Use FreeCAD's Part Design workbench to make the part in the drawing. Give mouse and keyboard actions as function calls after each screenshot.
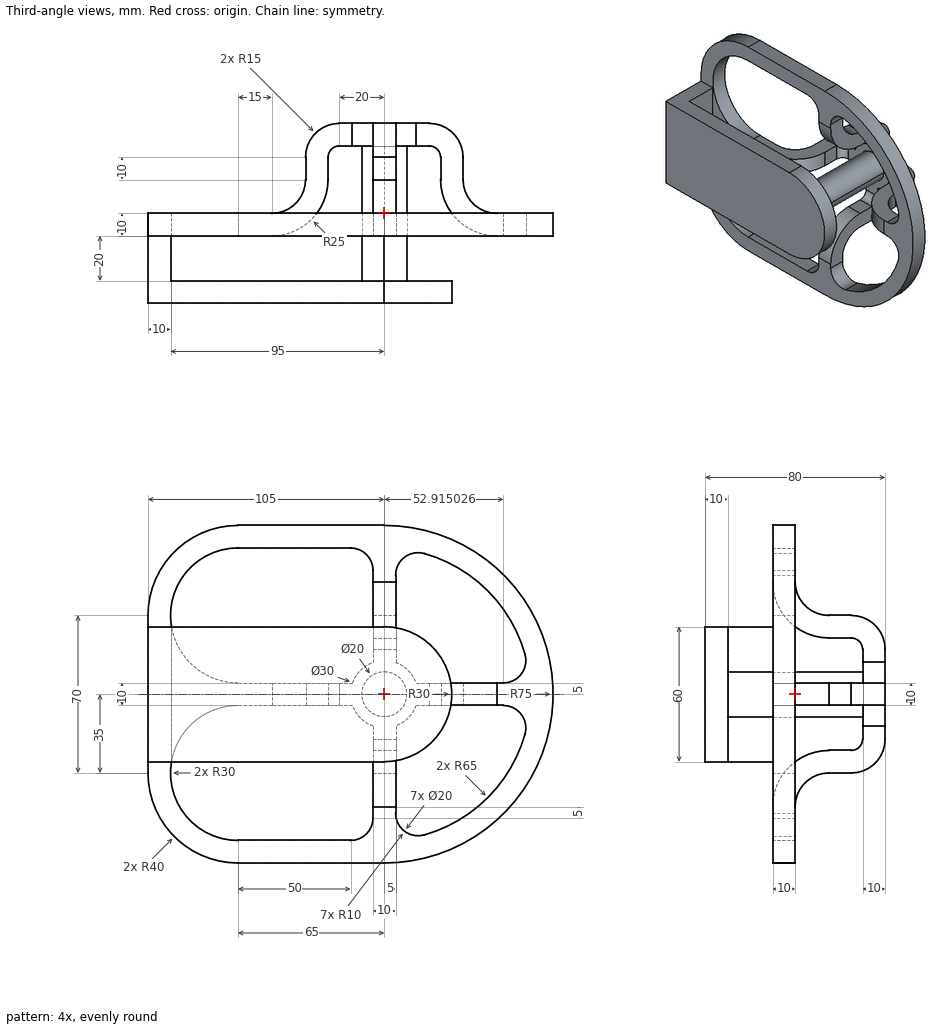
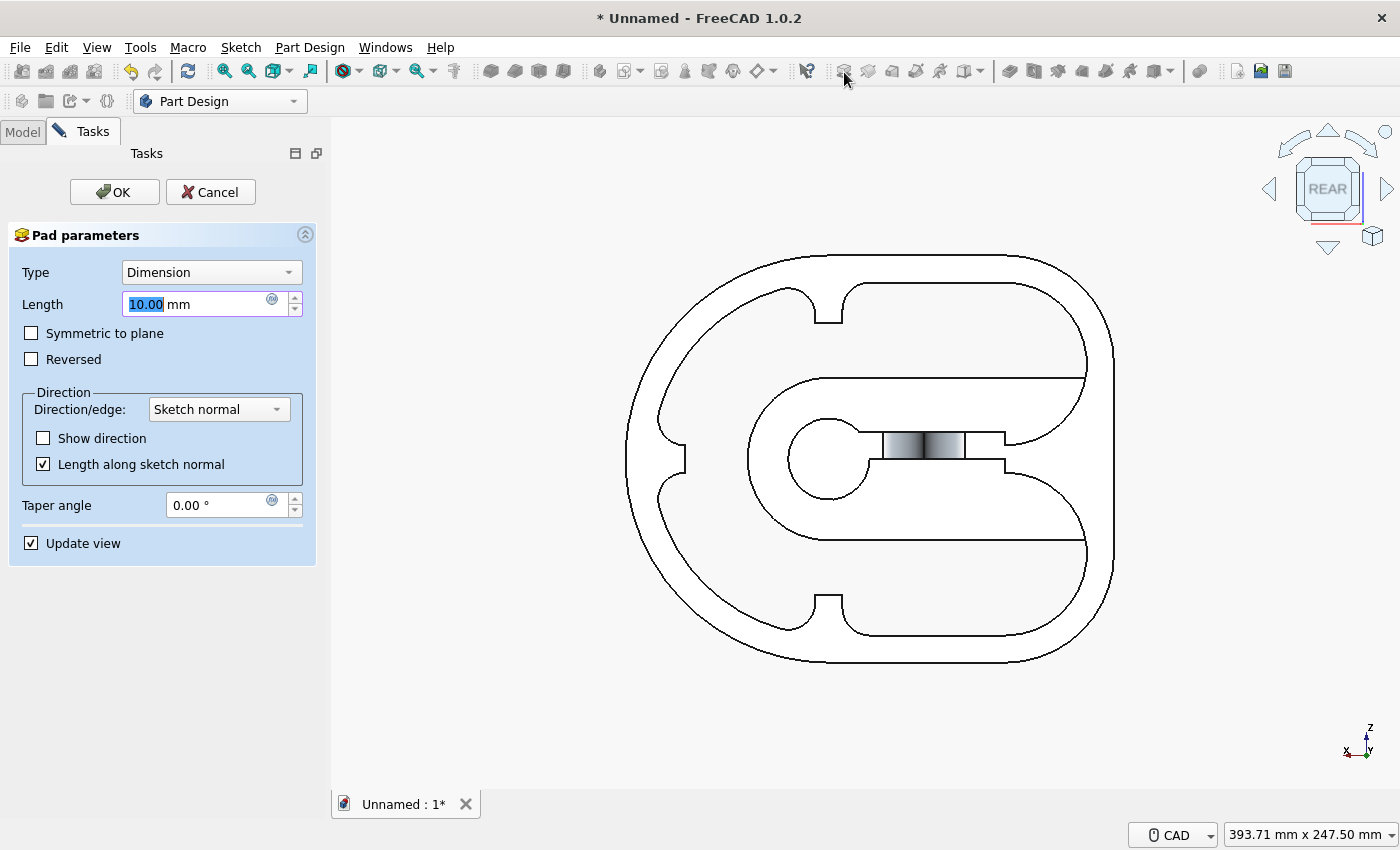
text(10)
key(Tab)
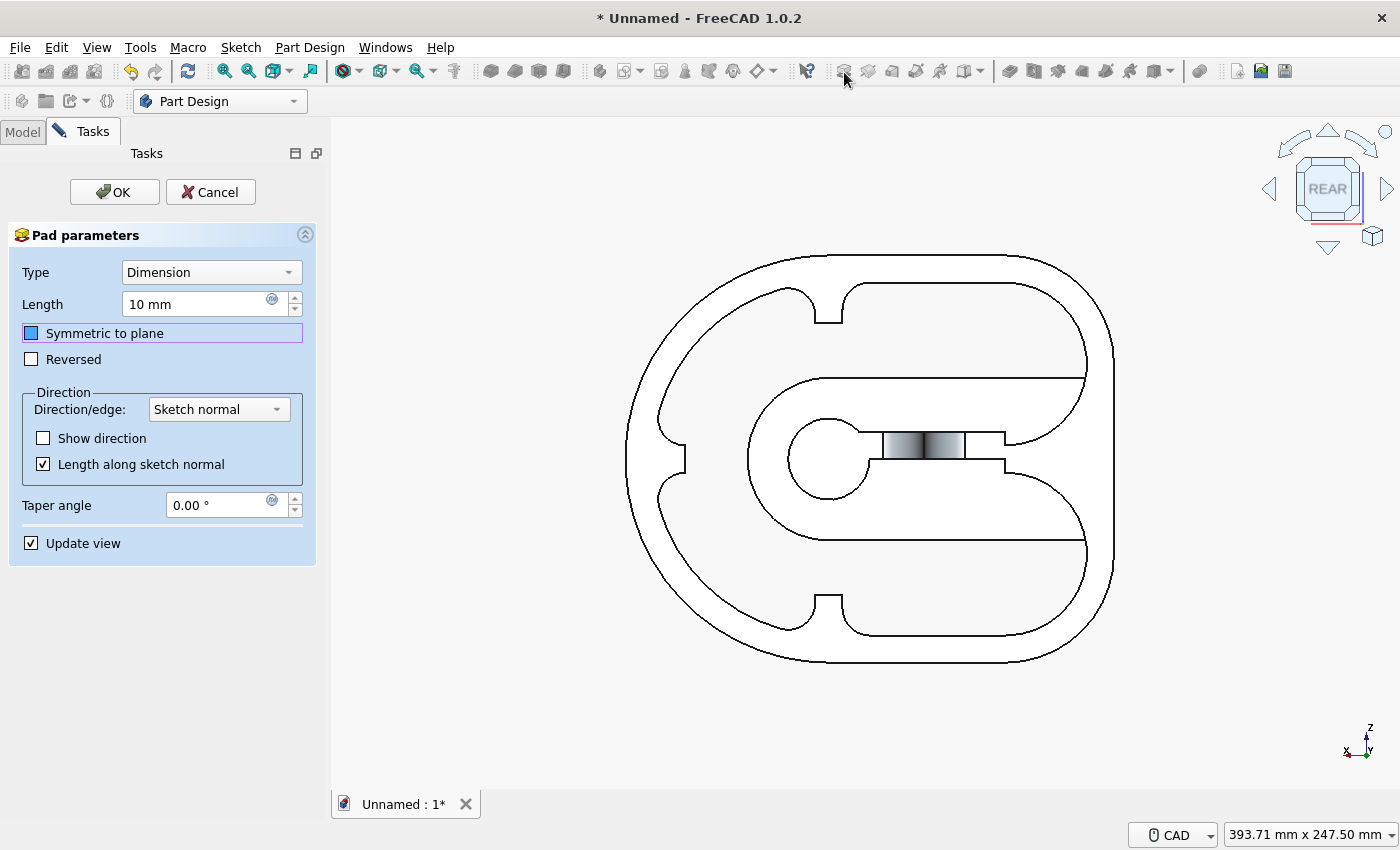
click(30, 333)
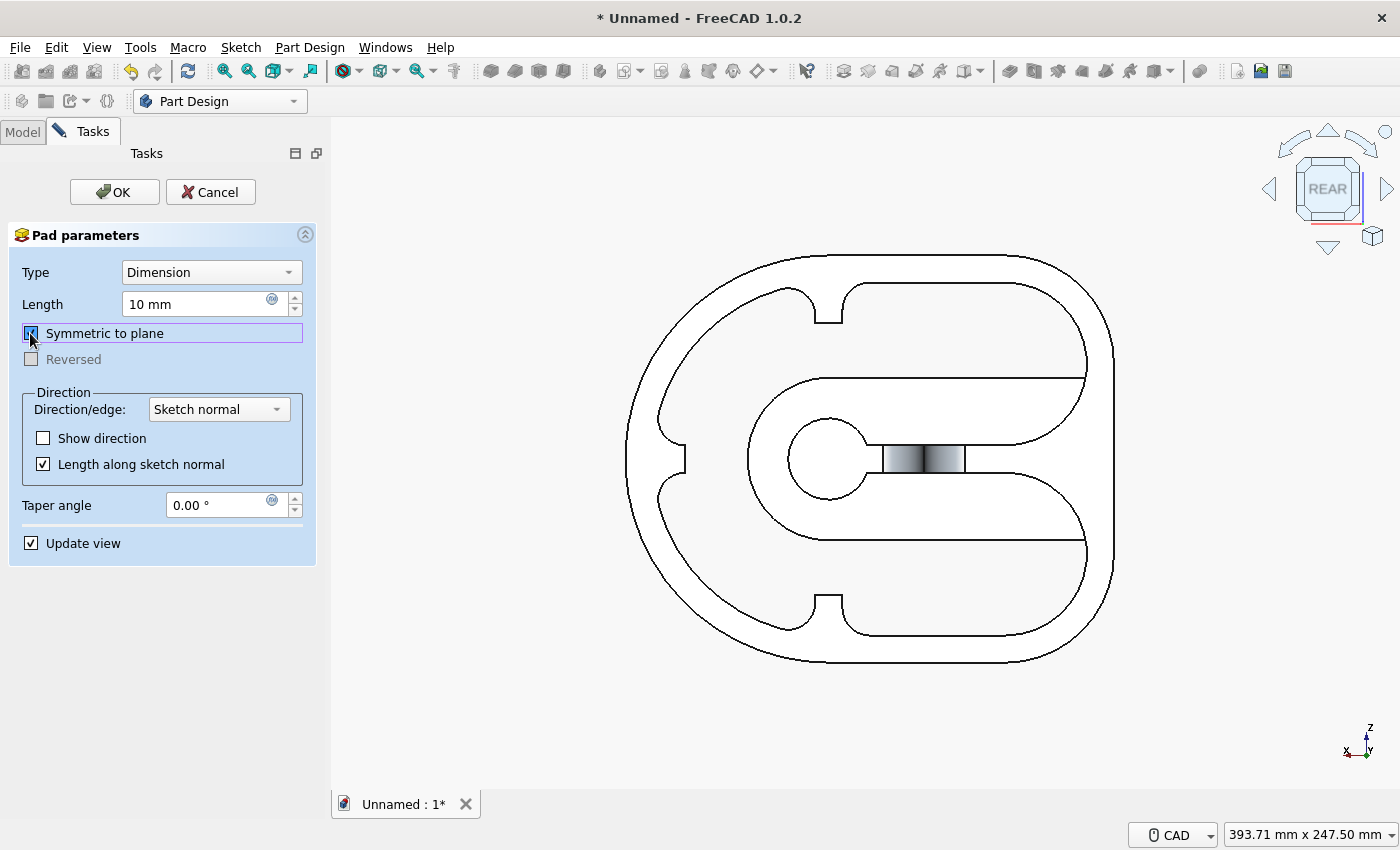
click(115, 192)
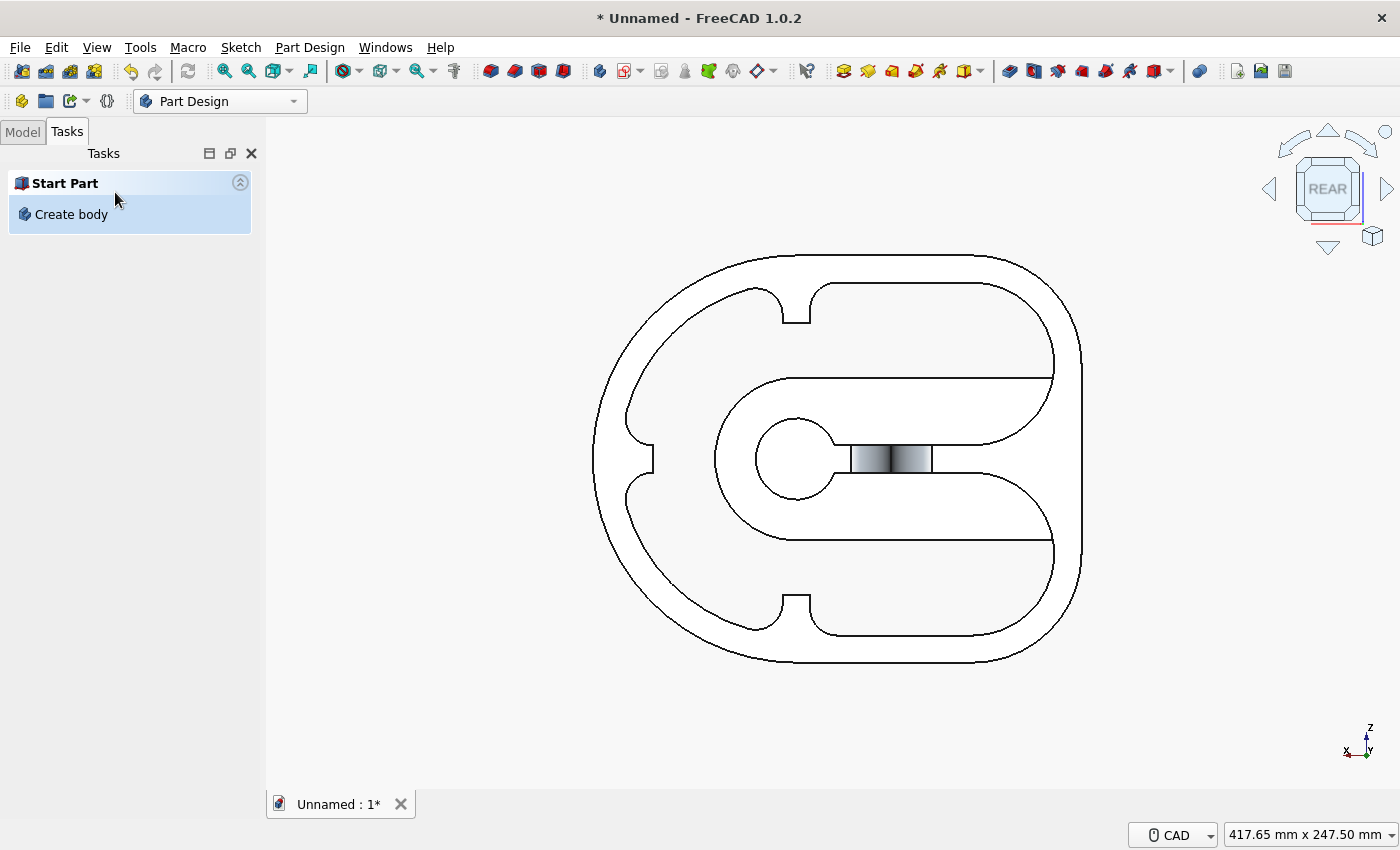
click(23, 131)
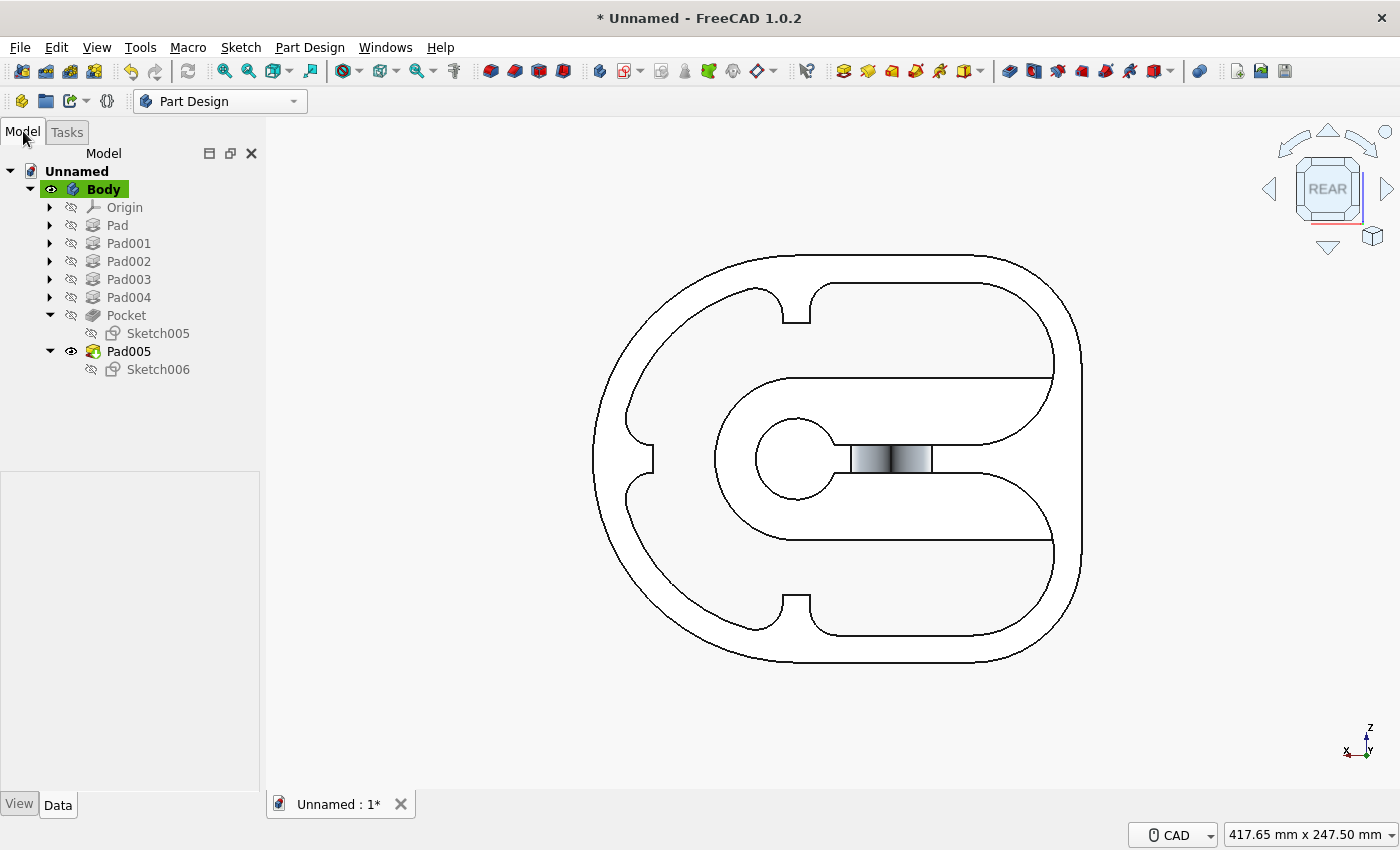
click(116, 351)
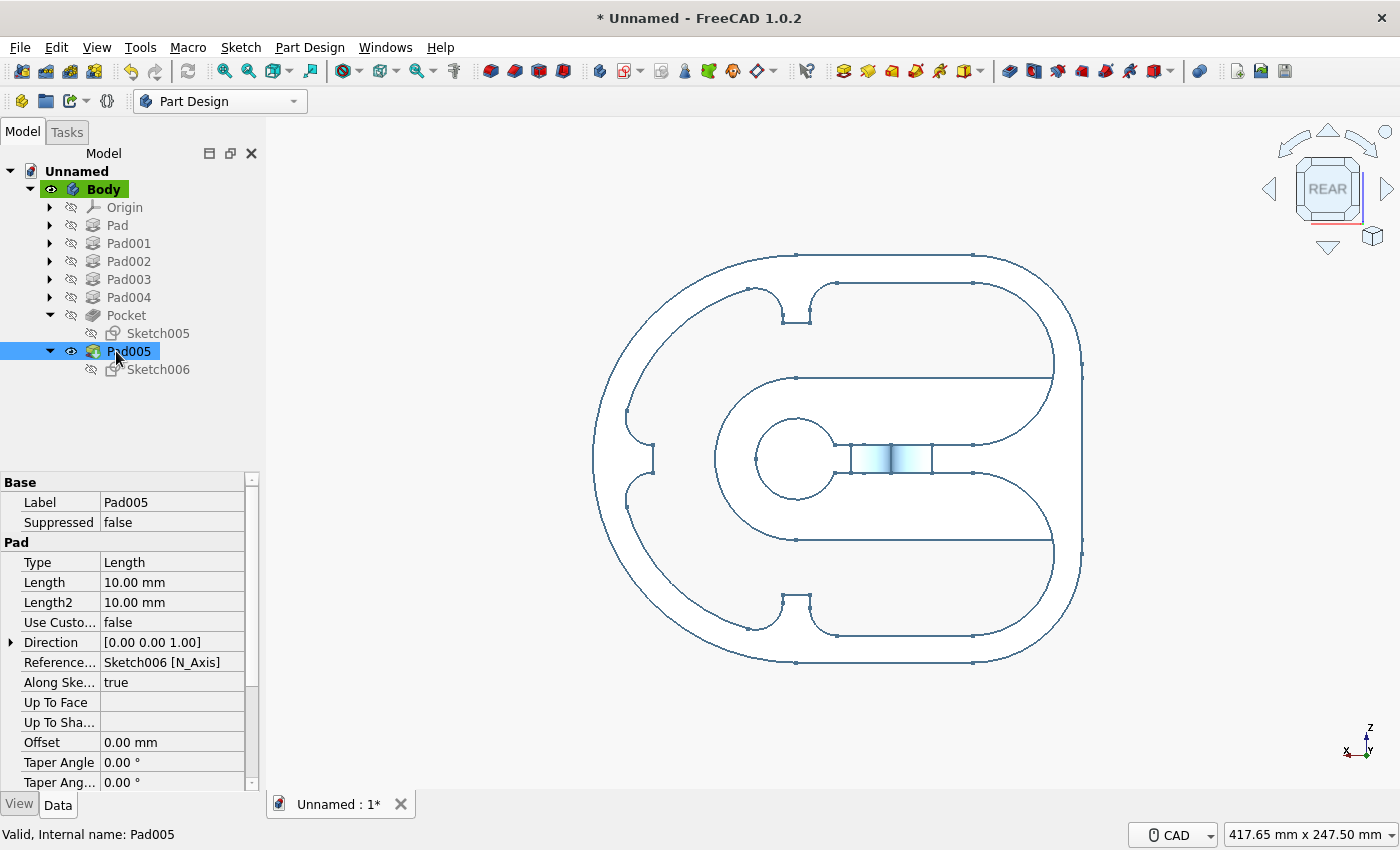
click(70, 72)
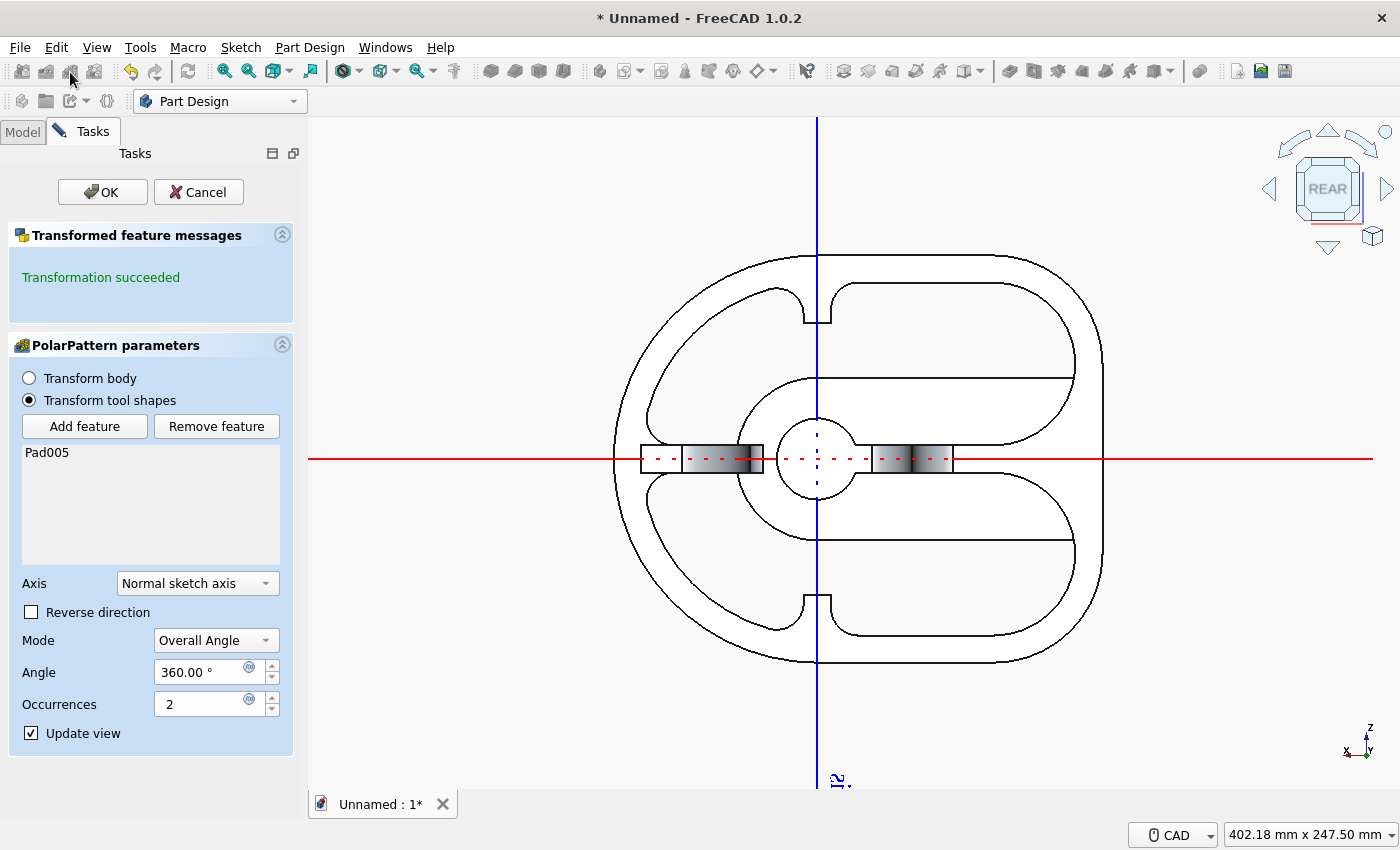
click(198, 584)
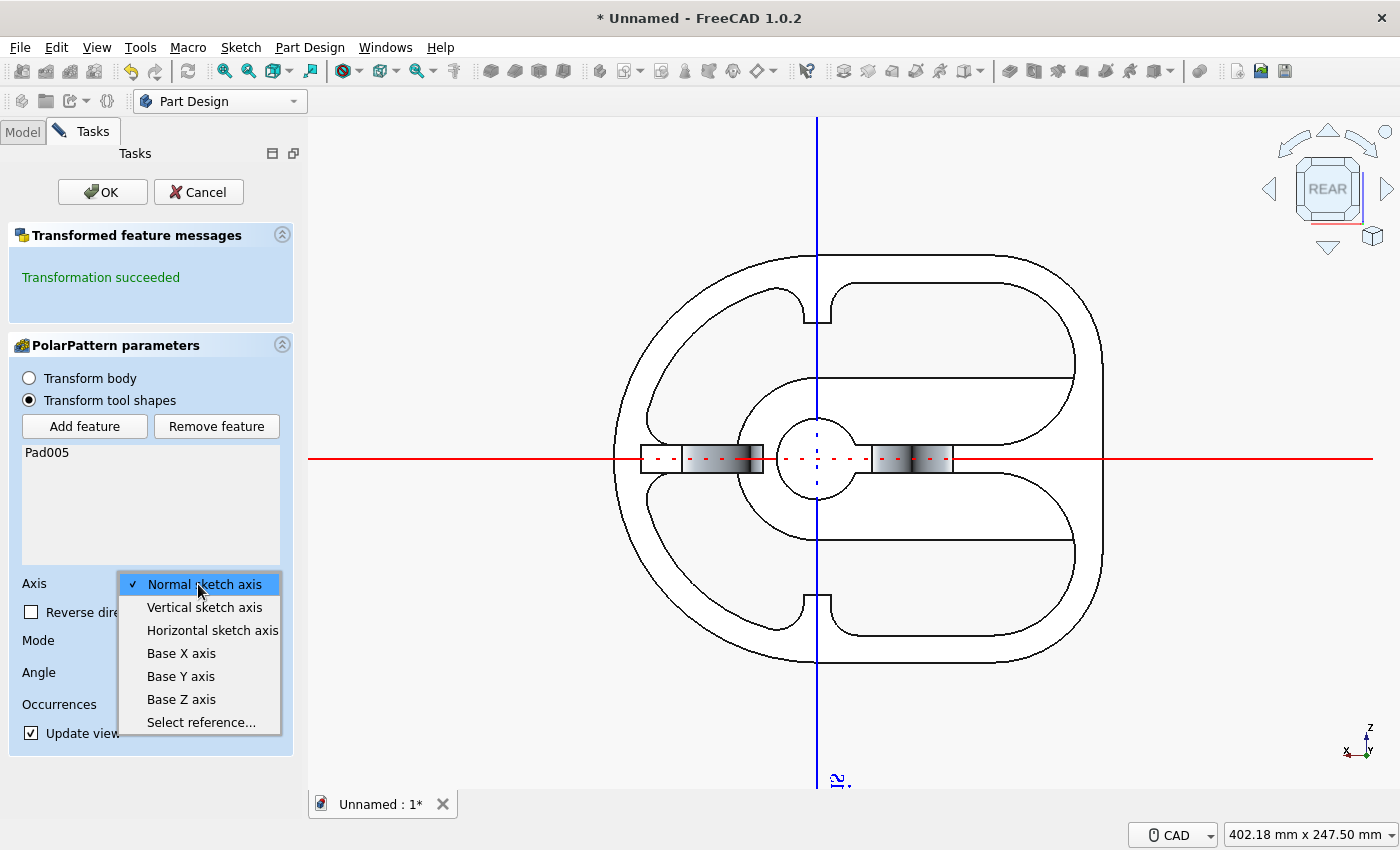
click(198, 676)